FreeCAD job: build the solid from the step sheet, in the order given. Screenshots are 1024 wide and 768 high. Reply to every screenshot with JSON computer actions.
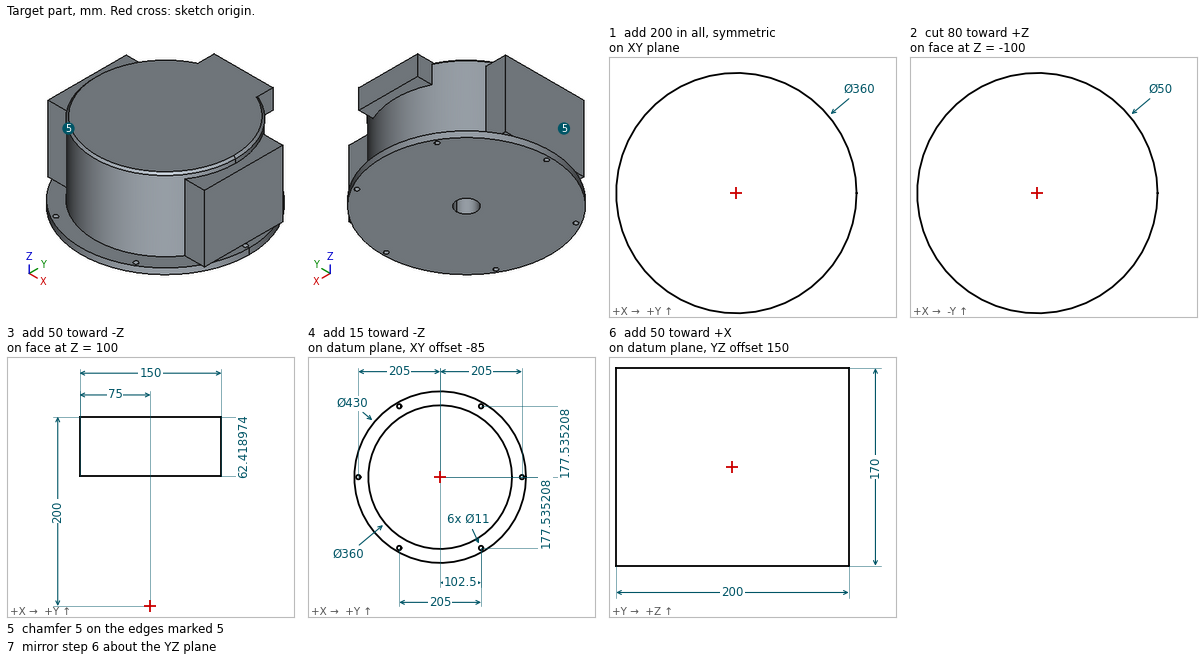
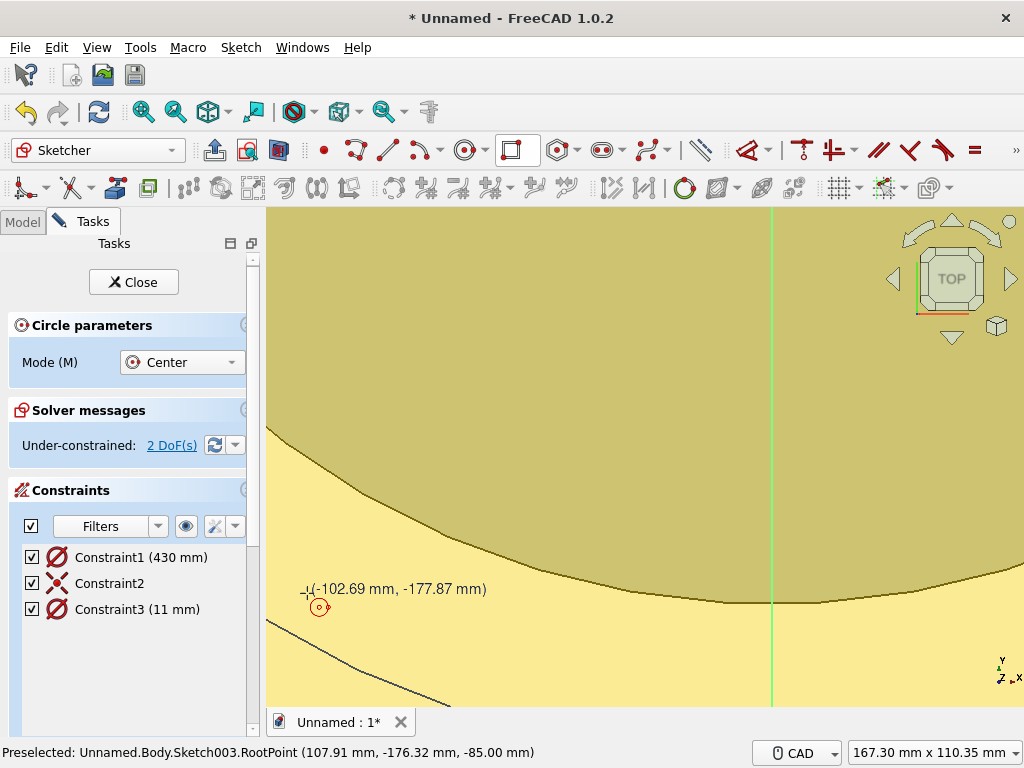
{"action": "left_click", "coordinate": [308, 593]}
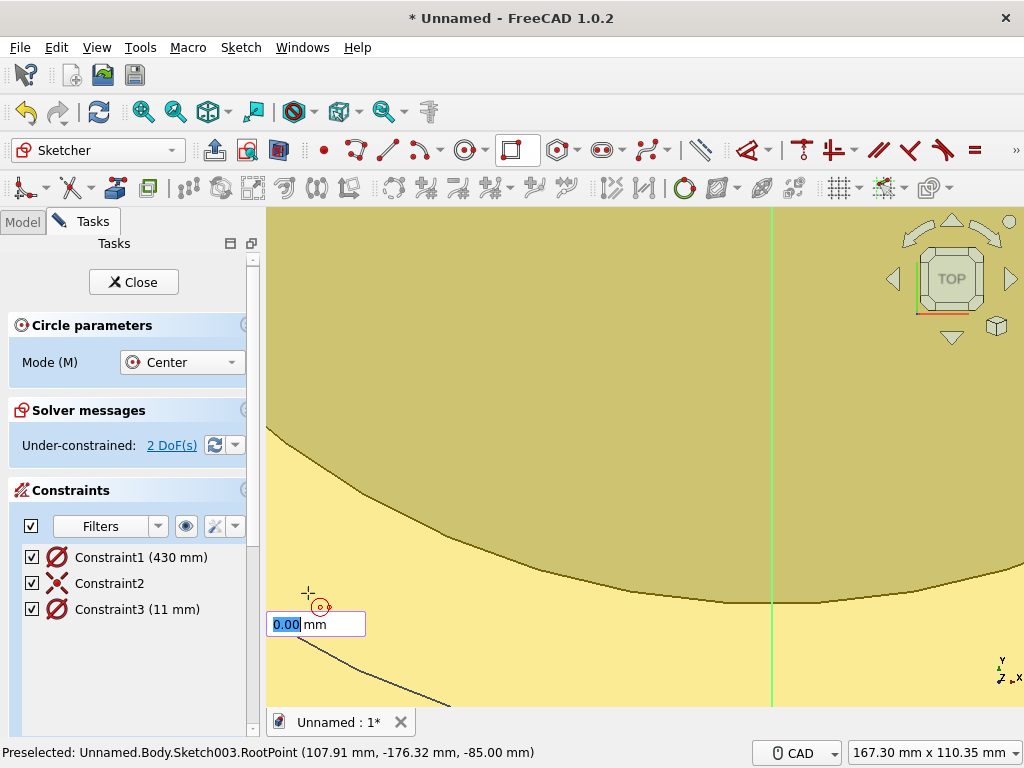
{"action": "scroll", "coordinate": [538, 589], "scroll_direction": "down", "scroll_amount": 9}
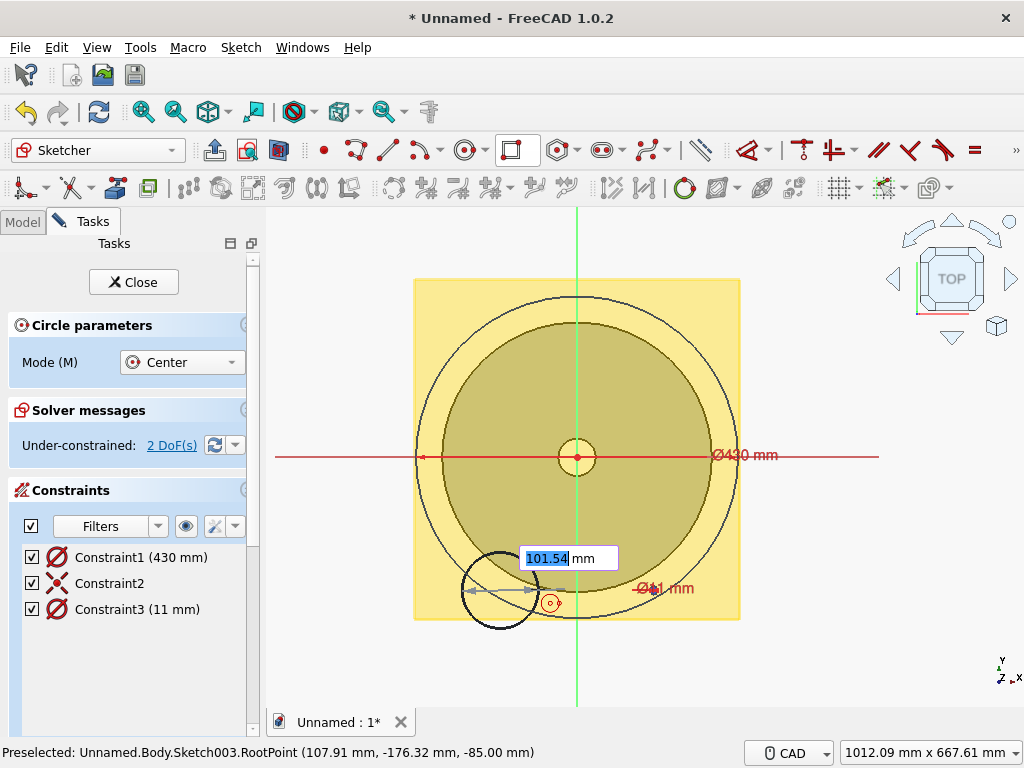
{"action": "scroll", "coordinate": [503, 587], "scroll_direction": "up", "scroll_amount": 2}
{"action": "mouse_move", "coordinate": [503, 587]}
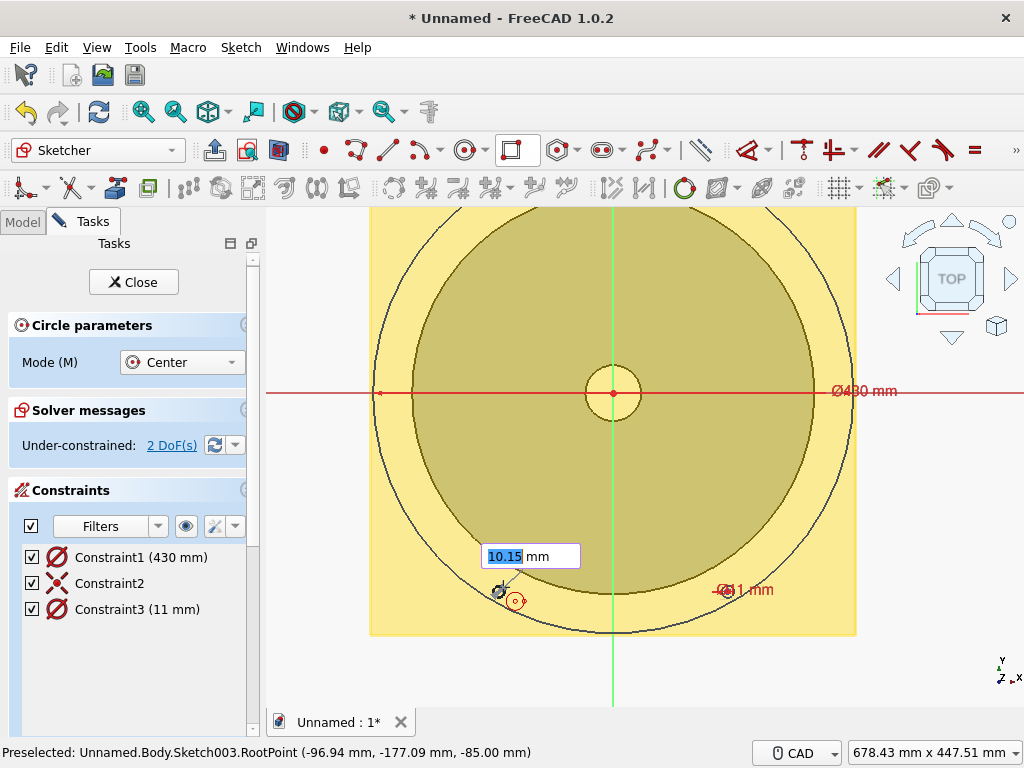
{"action": "type", "text": "11"}
{"action": "key", "text": "Return"}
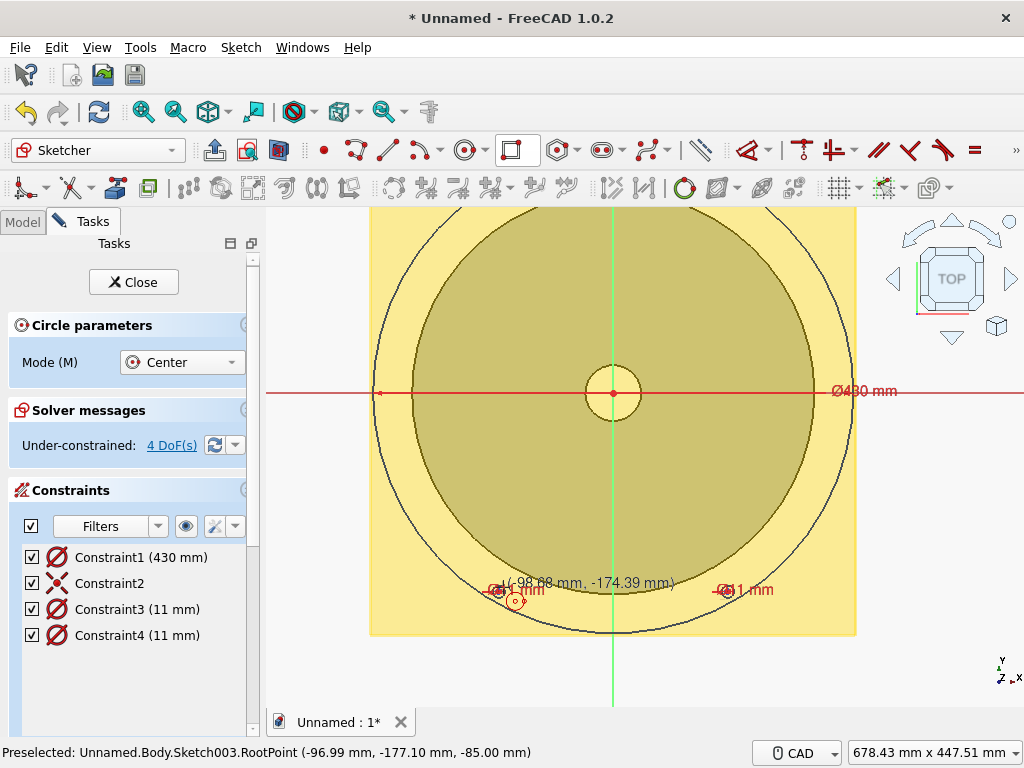
{"action": "scroll", "coordinate": [842, 393], "scroll_direction": "up", "scroll_amount": 7}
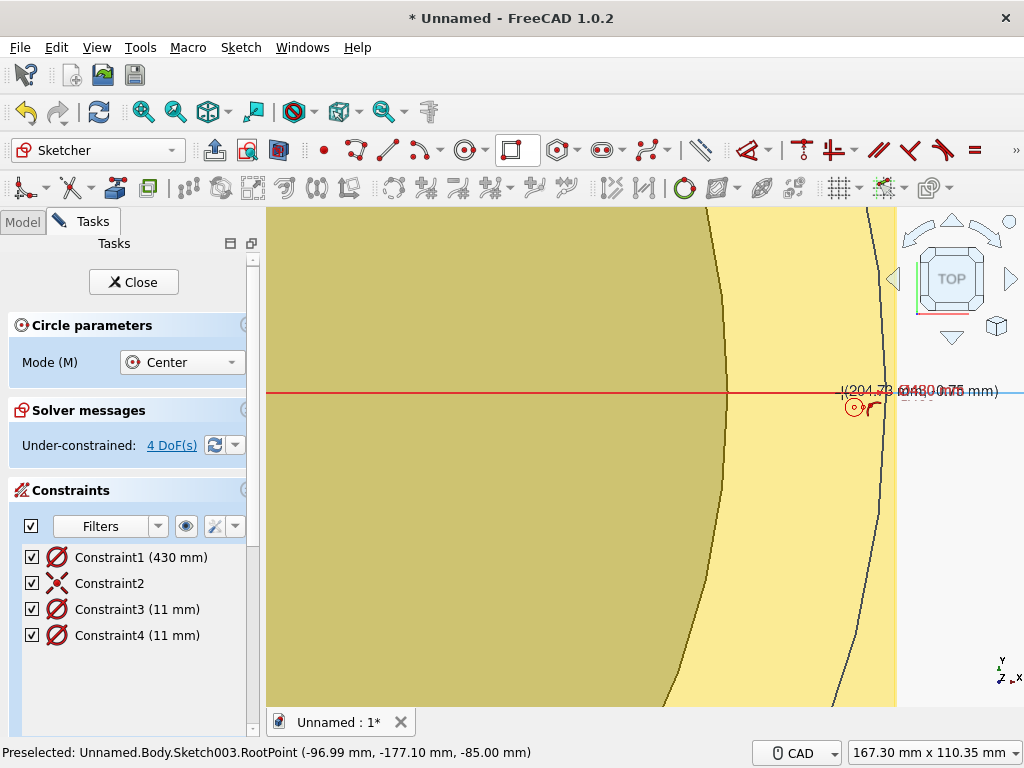
{"action": "left_click", "coordinate": [841, 393]}
{"action": "mouse_move", "coordinate": [858, 375]}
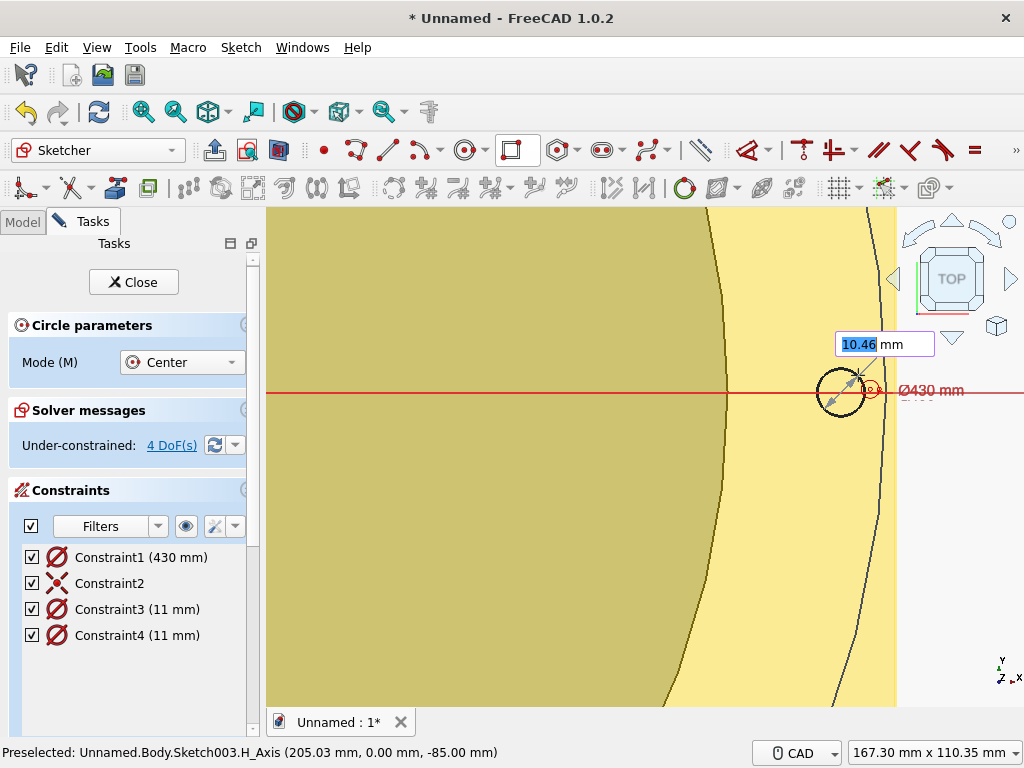
{"action": "type", "text": "11"}
{"action": "key", "text": "Return"}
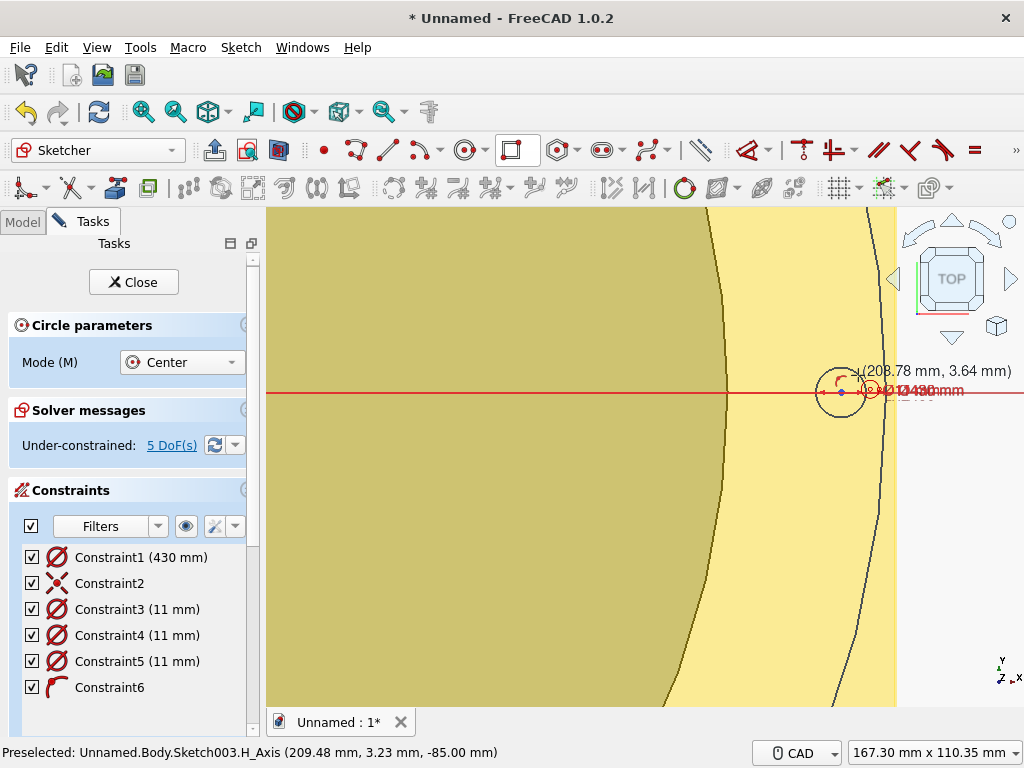
{"action": "scroll", "coordinate": [708, 470], "scroll_direction": "down", "scroll_amount": 9}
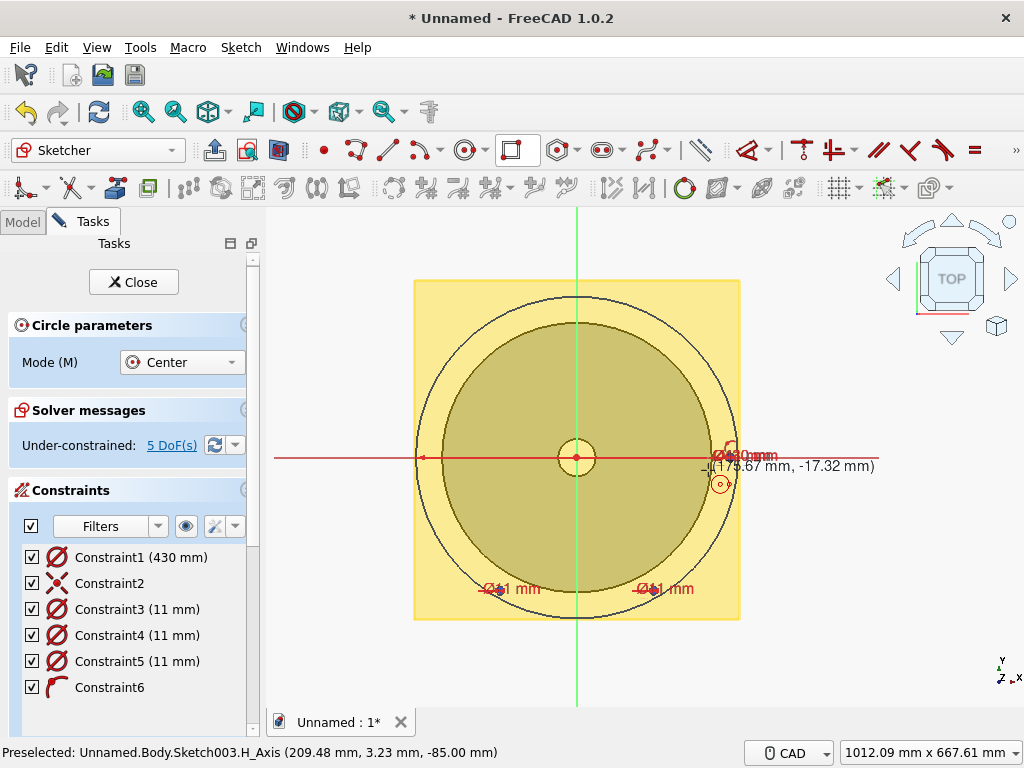
{"action": "scroll", "coordinate": [654, 325], "scroll_direction": "up", "scroll_amount": 9}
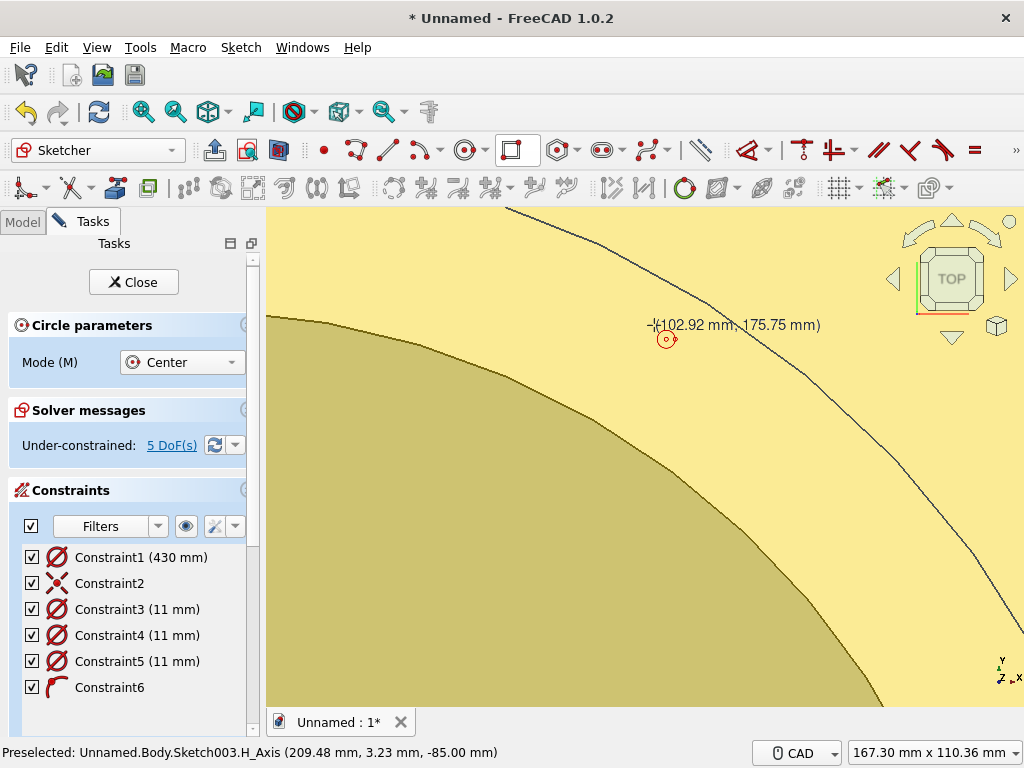
{"action": "left_click", "coordinate": [650, 322]}
{"action": "mouse_move", "coordinate": [667, 304]}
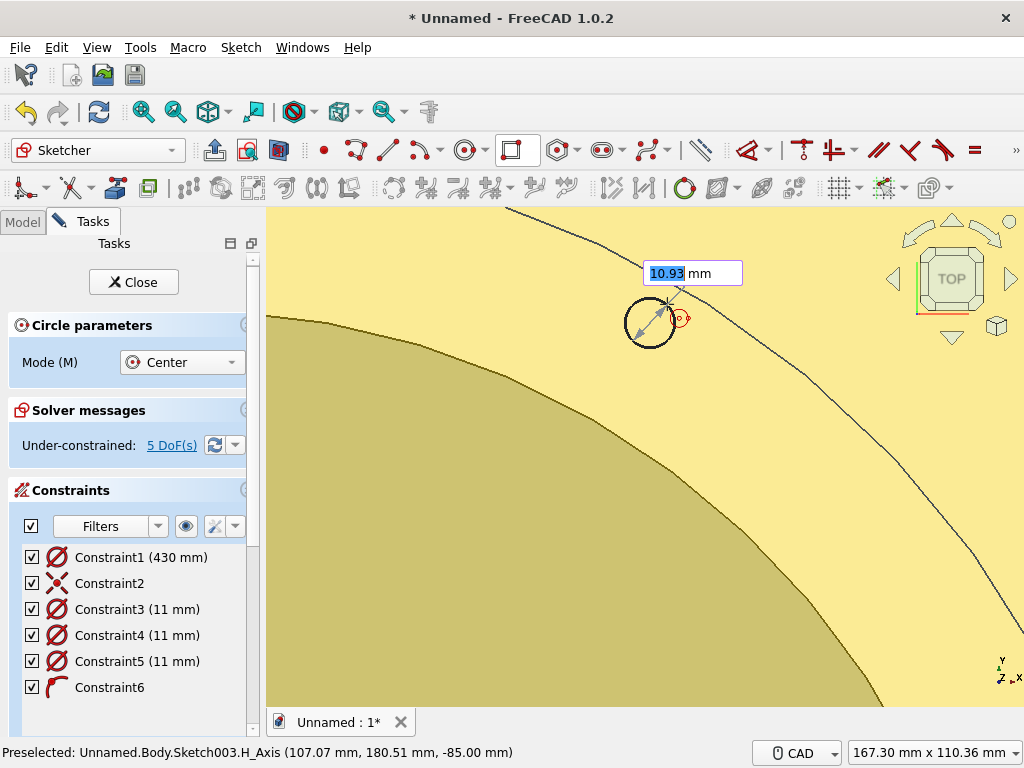
{"action": "type", "text": "11"}
{"action": "key", "text": "Return"}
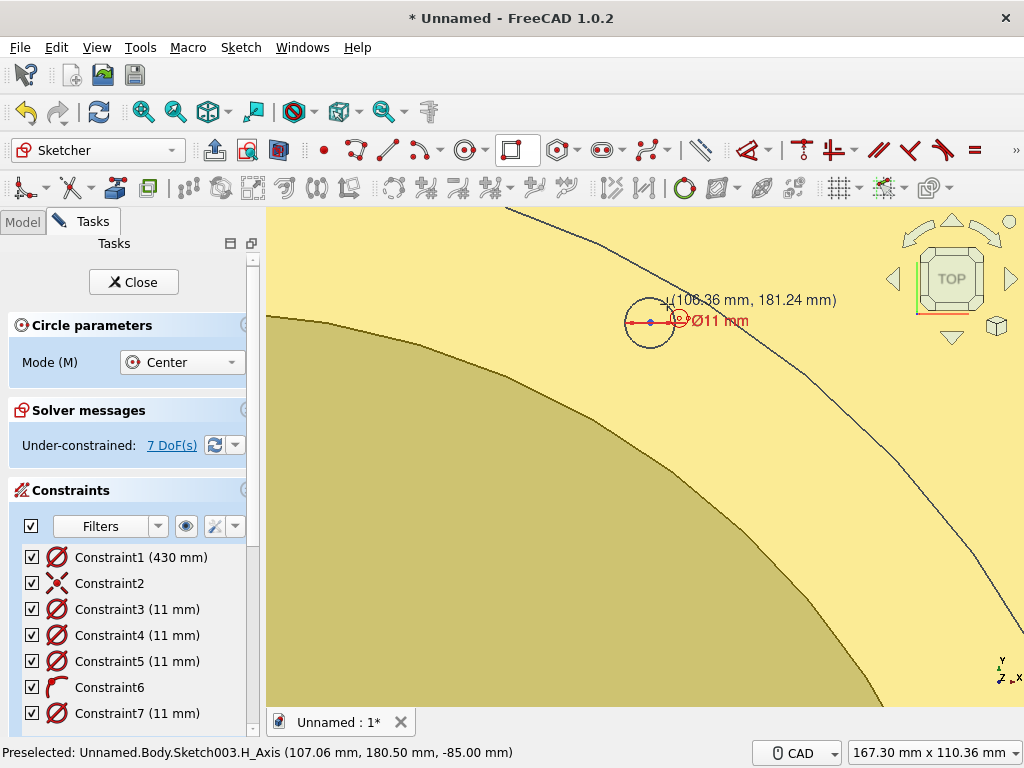
{"action": "scroll", "coordinate": [654, 324], "scroll_direction": "down", "scroll_amount": 9}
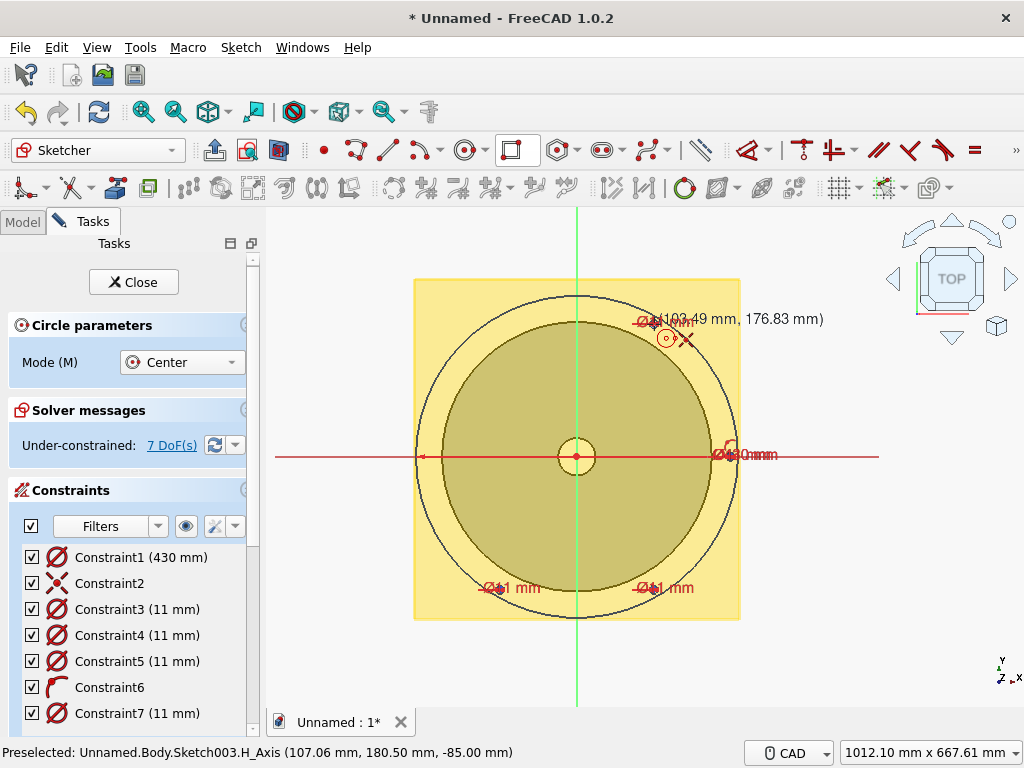
{"action": "left_click", "coordinate": [577, 457]}
{"action": "mouse_move", "coordinate": [672, 361]}